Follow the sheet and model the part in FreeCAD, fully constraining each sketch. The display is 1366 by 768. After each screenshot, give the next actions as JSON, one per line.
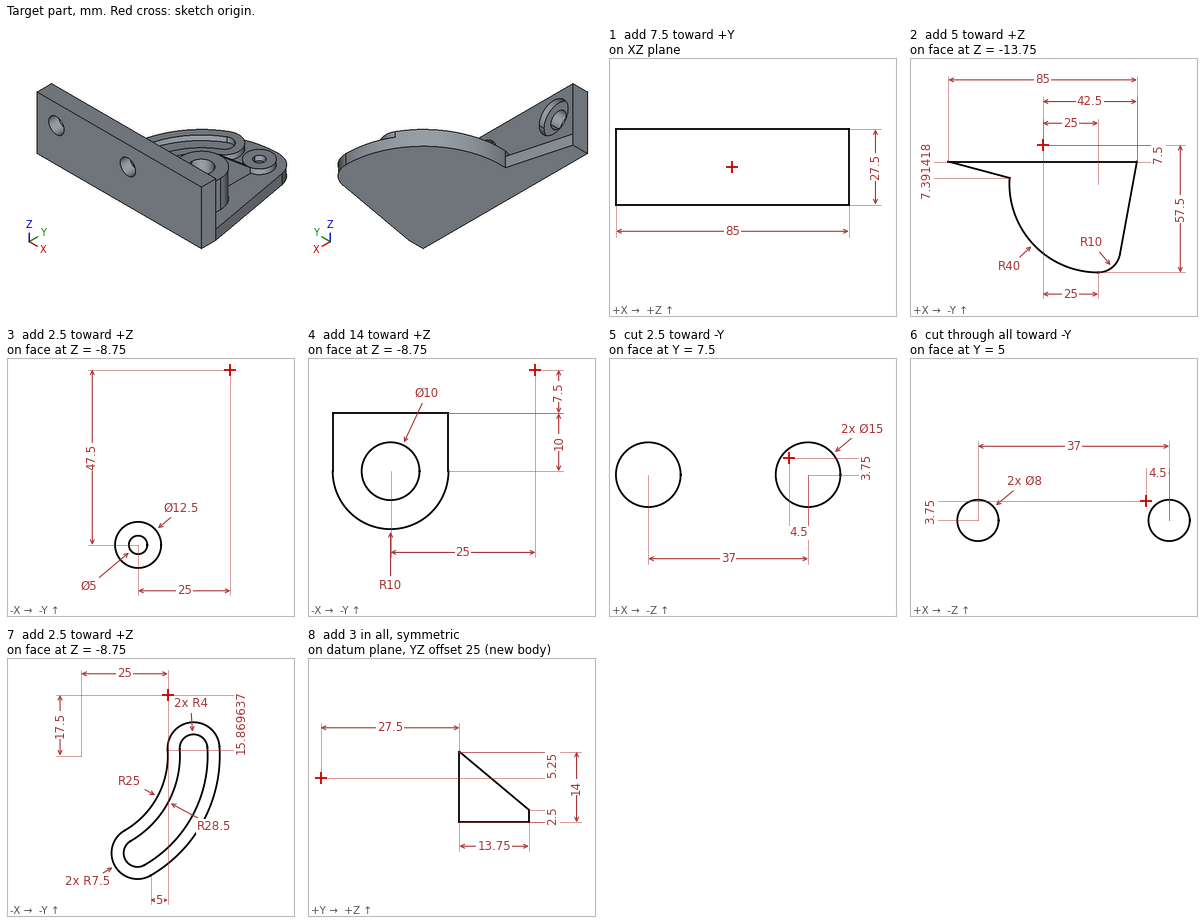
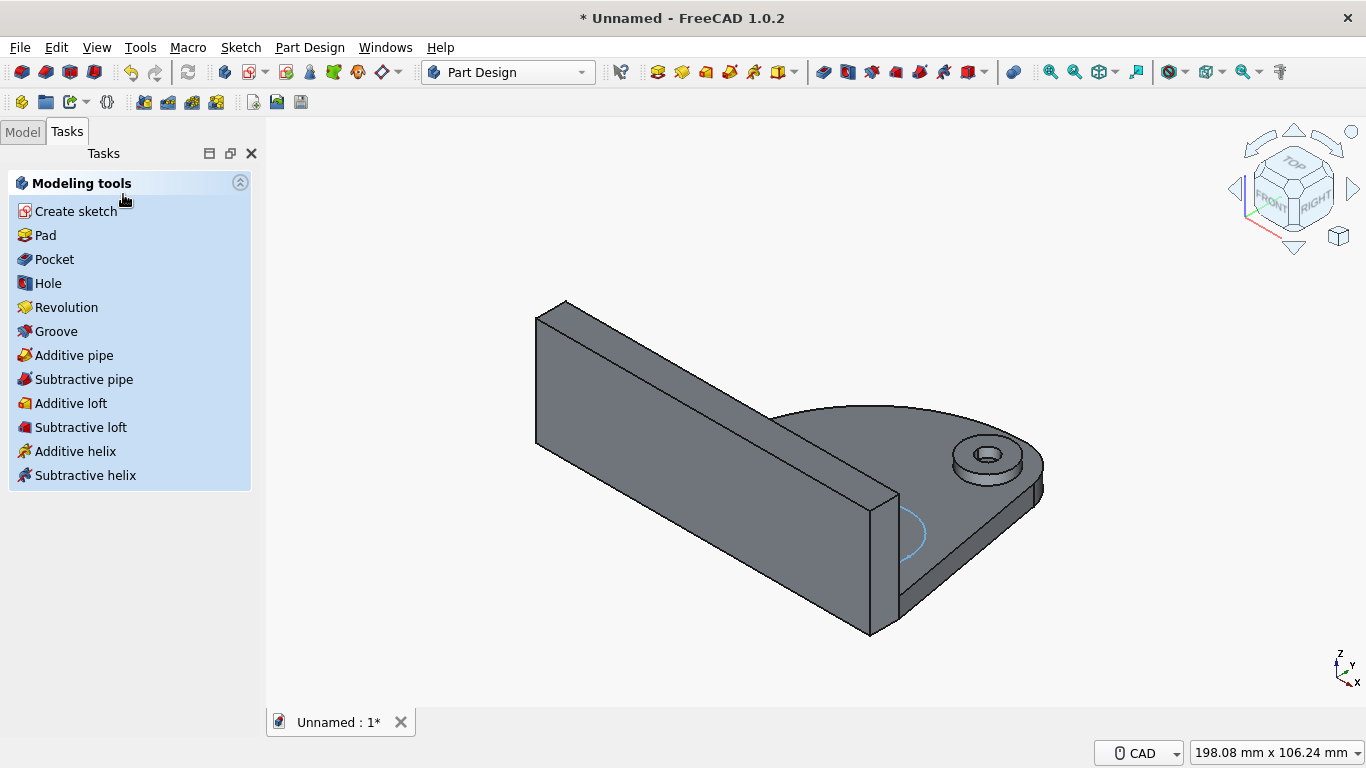
{"action": "left_click", "coordinate": [658, 72]}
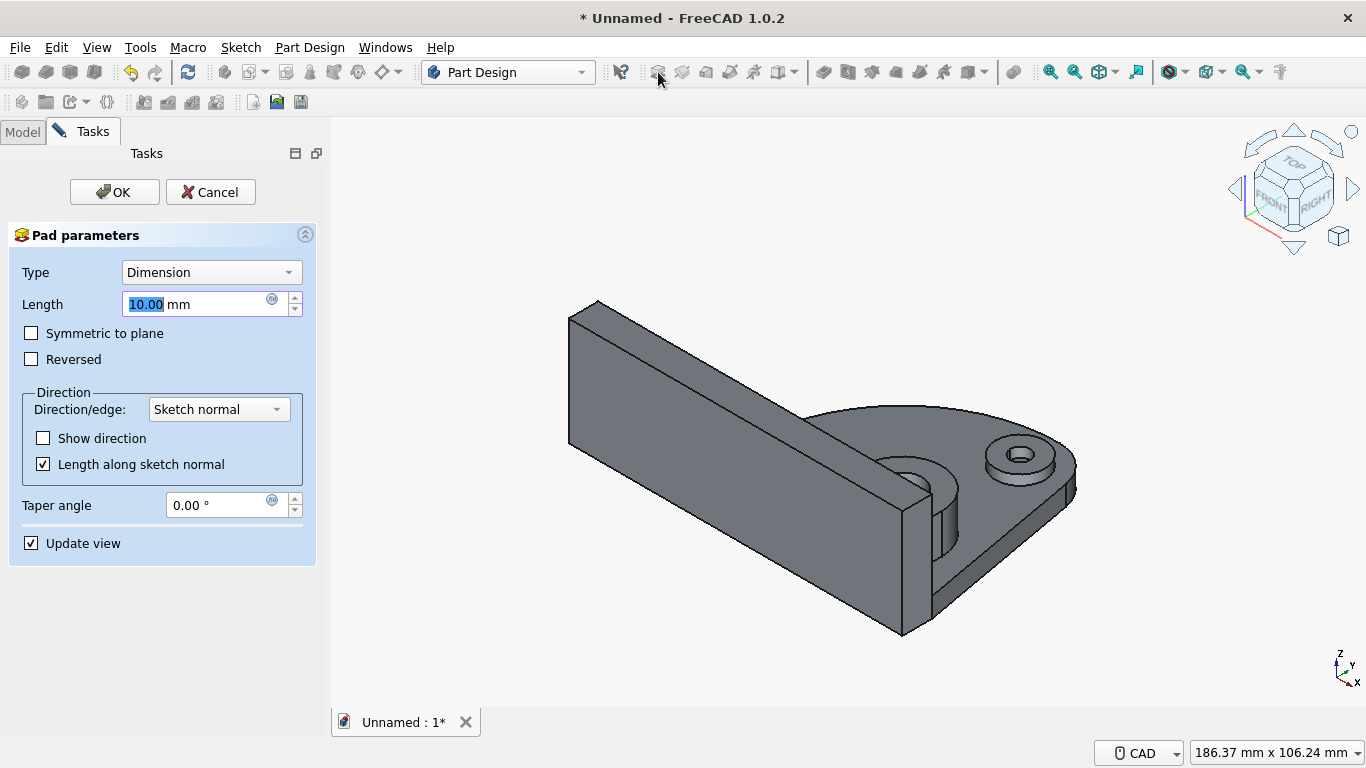
{"action": "type", "text": "14"}
{"action": "key", "text": "Tab"}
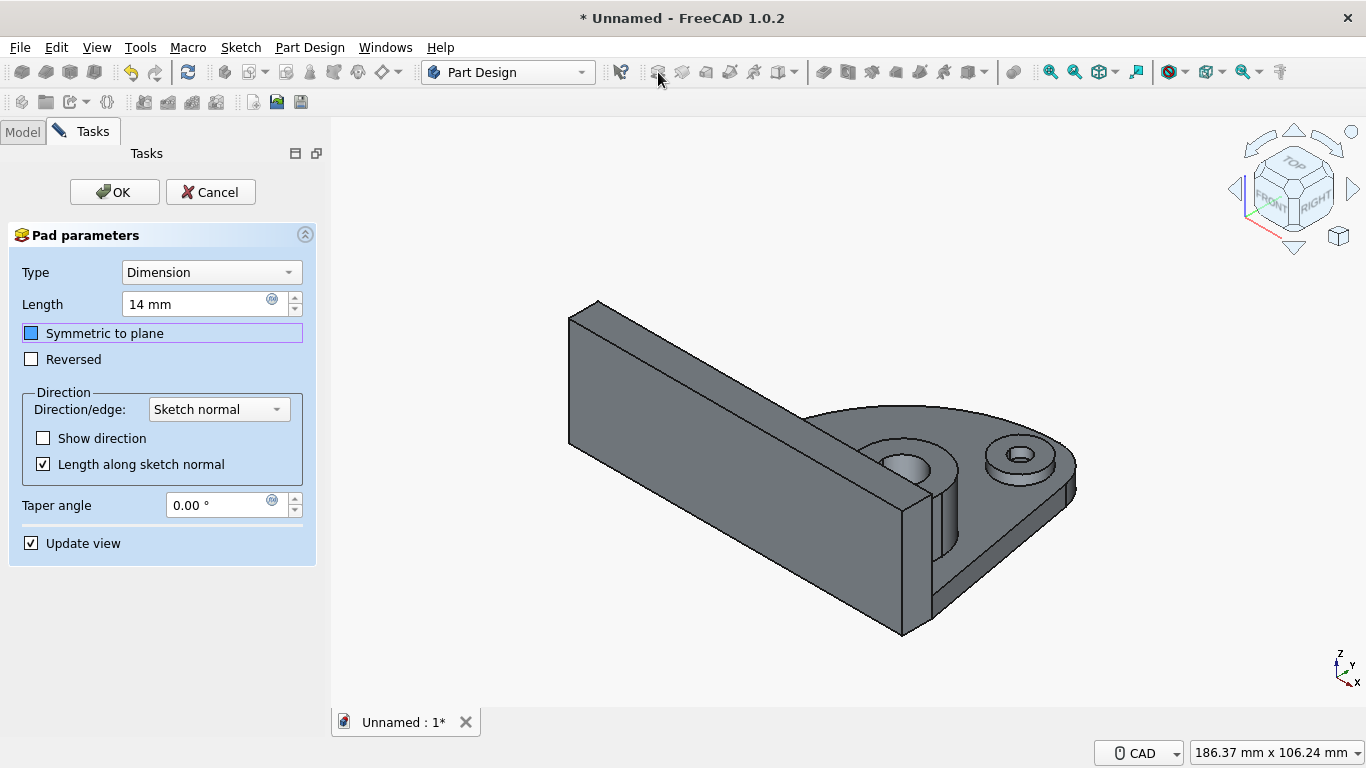
{"action": "left_click", "coordinate": [115, 192]}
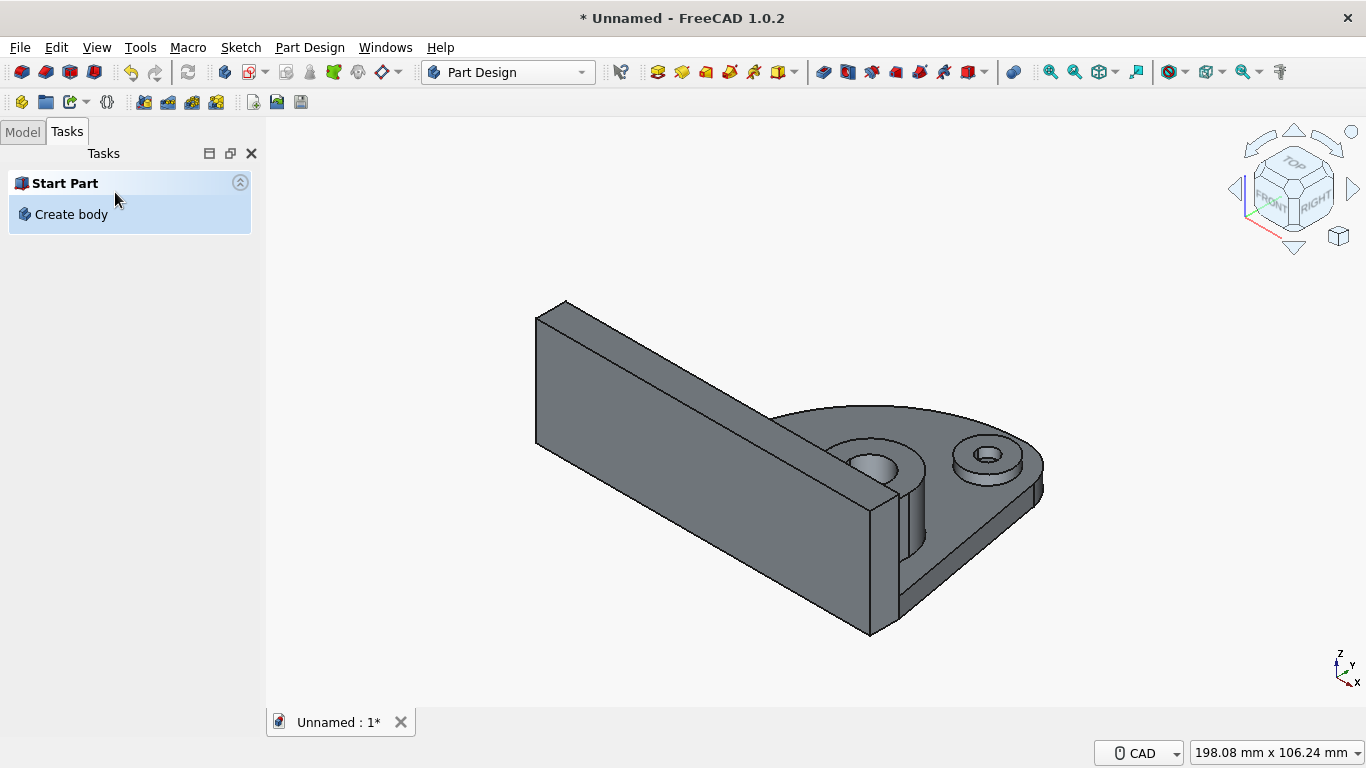
{"action": "key", "text": "4"}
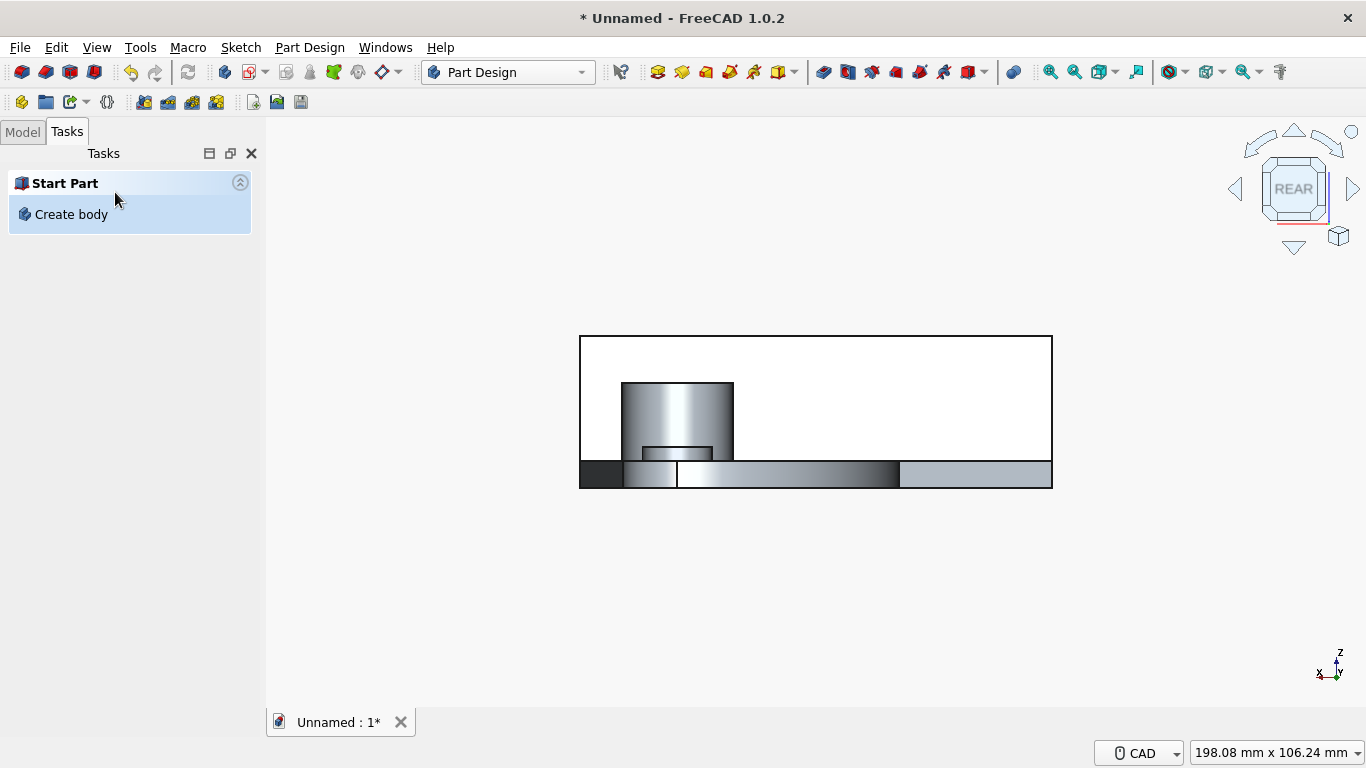
{"action": "left_click", "coordinate": [1052, 72]}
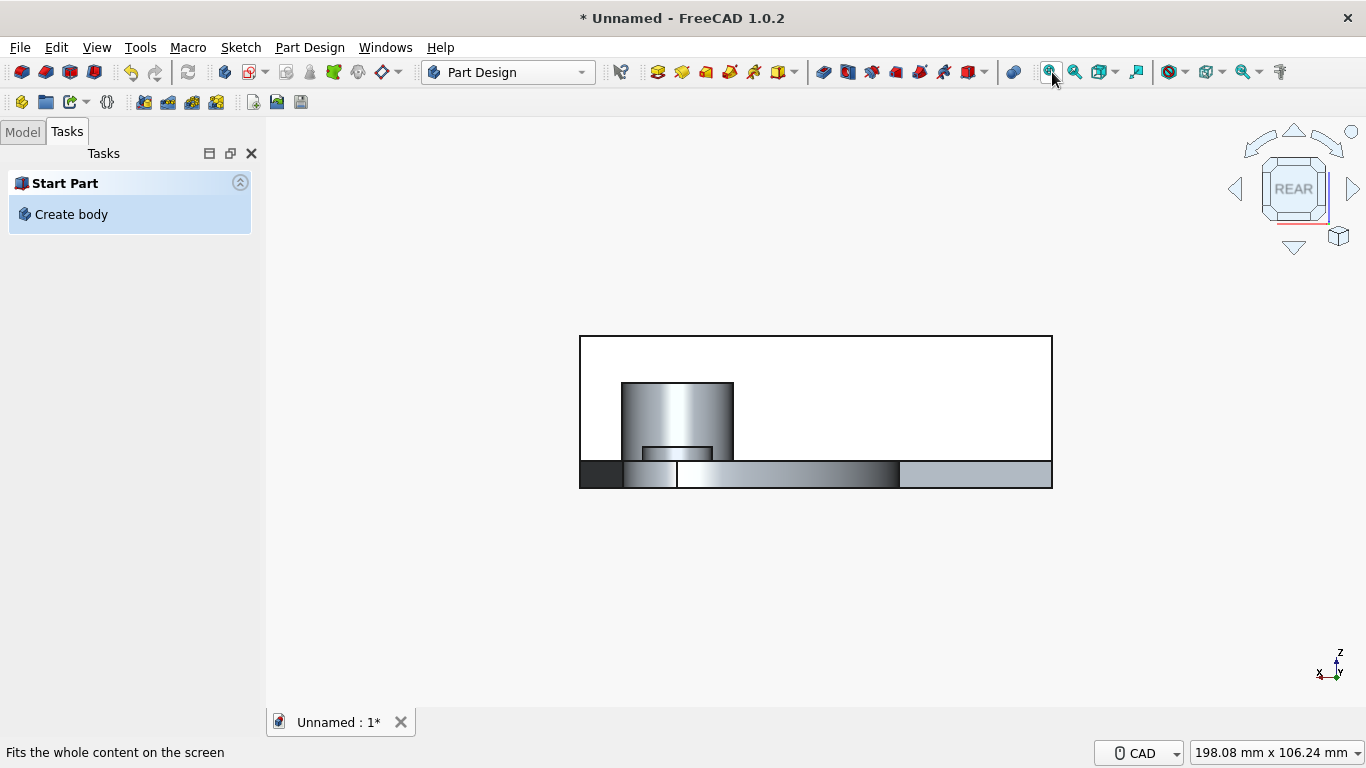
{"action": "left_click", "coordinate": [816, 397]}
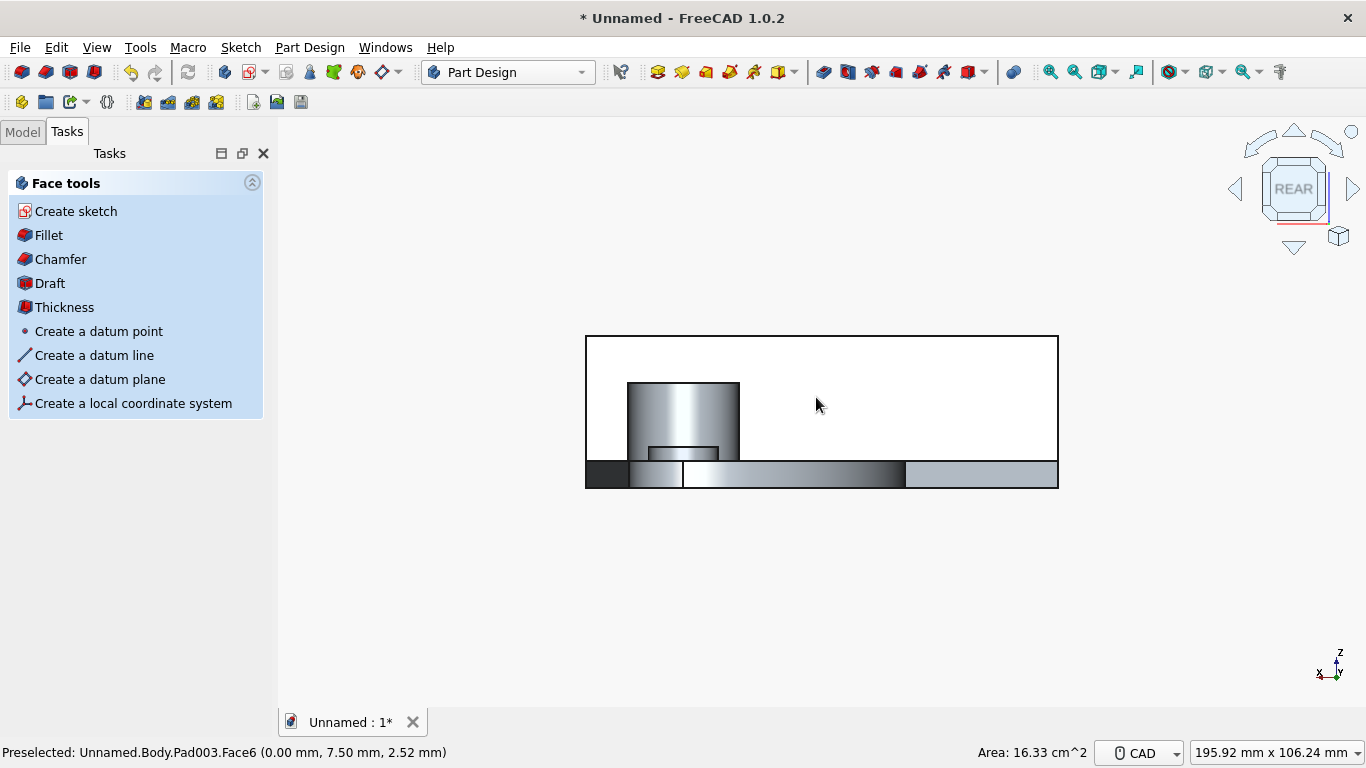
{"action": "left_click", "coordinate": [250, 72]}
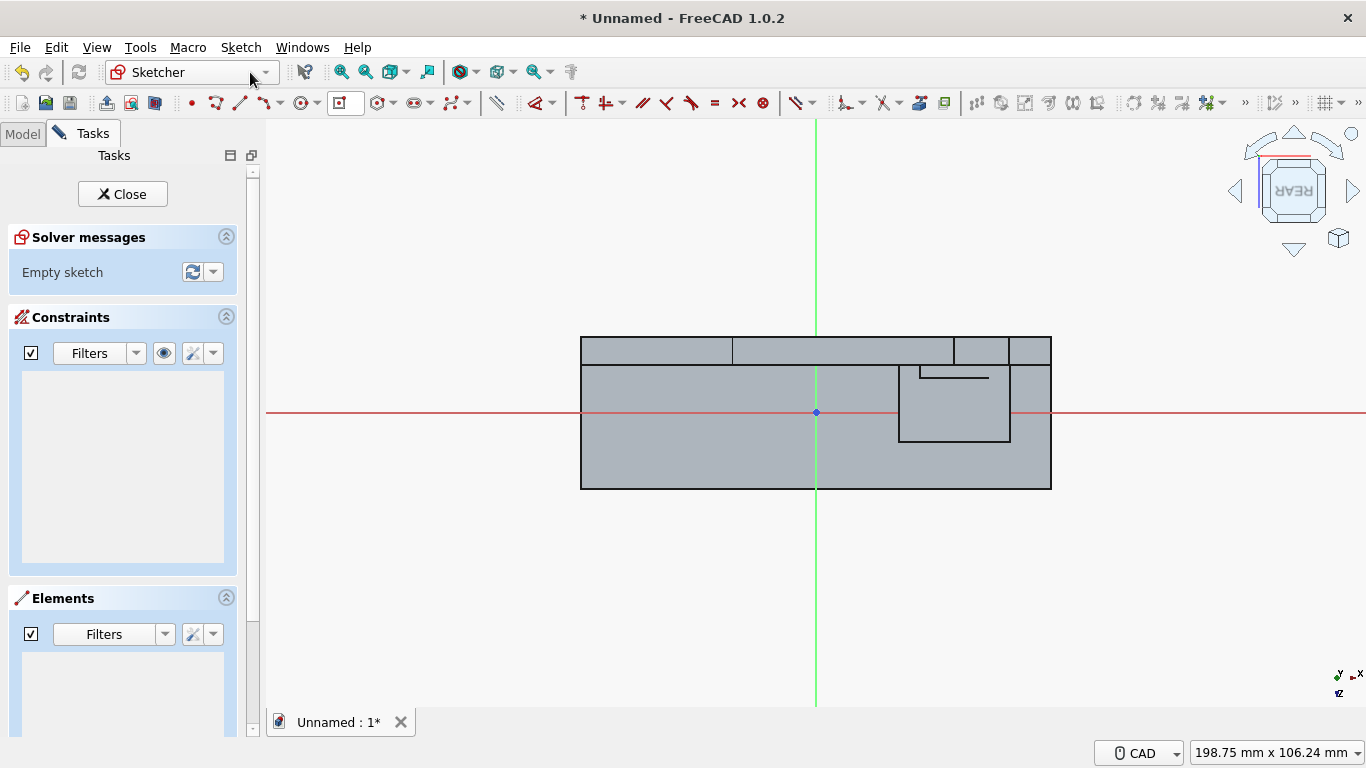
{"action": "scroll", "coordinate": [731, 451], "scroll_direction": "up", "scroll_amount": 4}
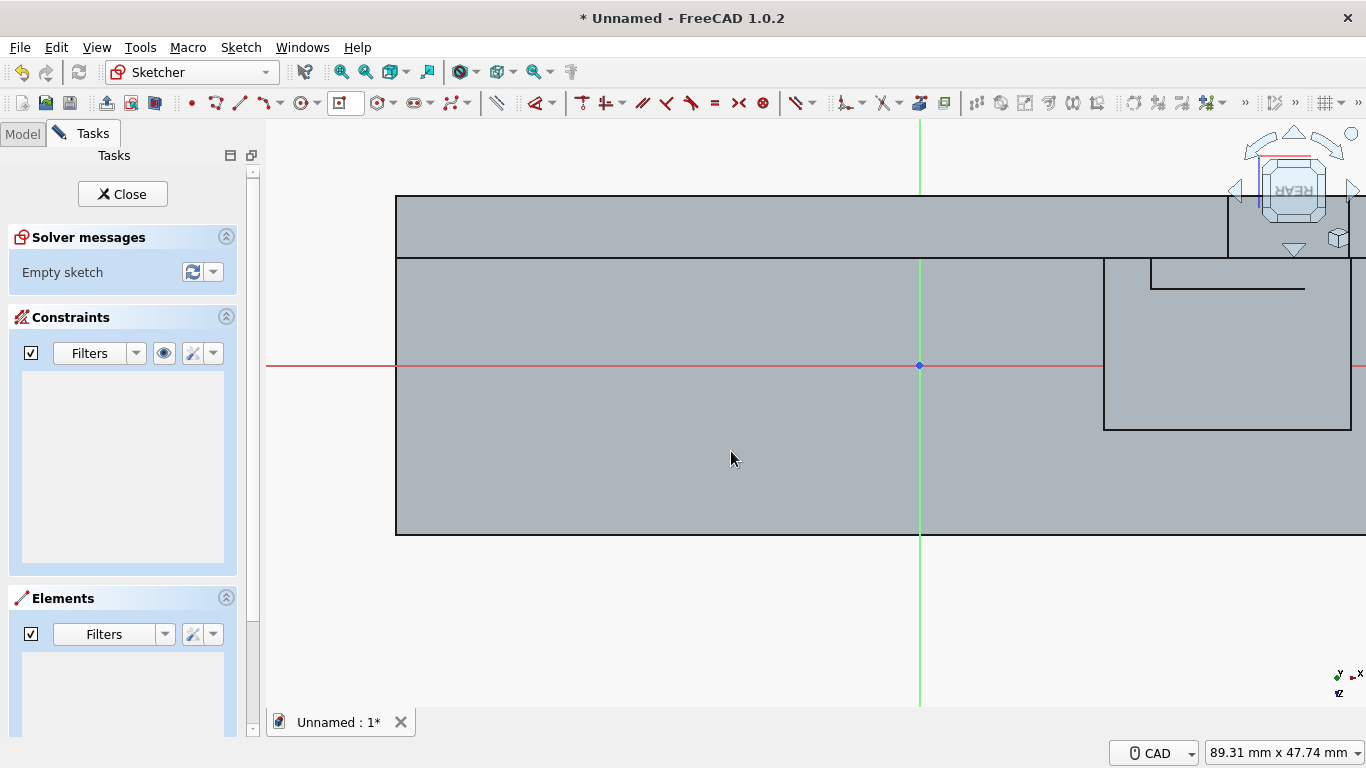
{"action": "left_click", "coordinate": [302, 104]}